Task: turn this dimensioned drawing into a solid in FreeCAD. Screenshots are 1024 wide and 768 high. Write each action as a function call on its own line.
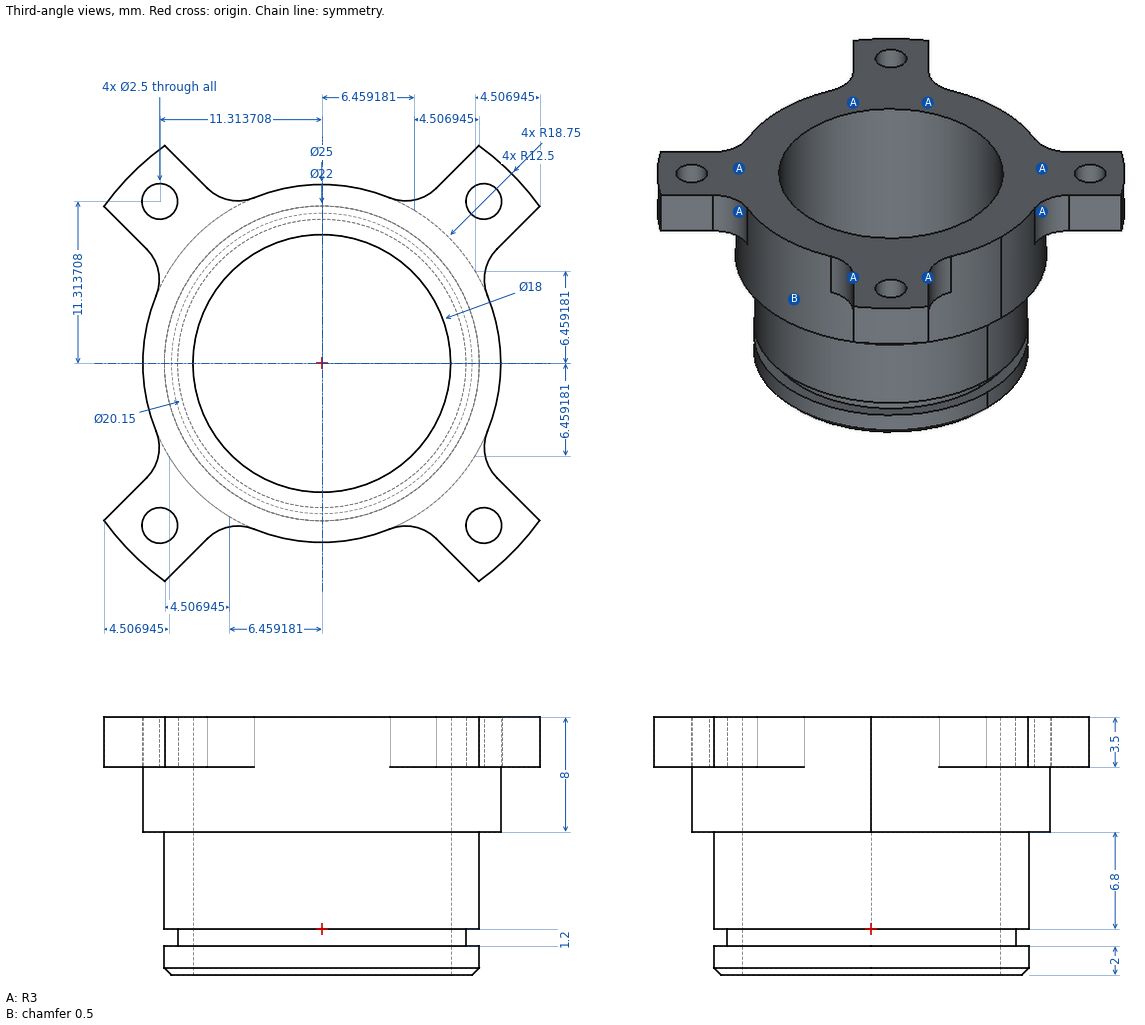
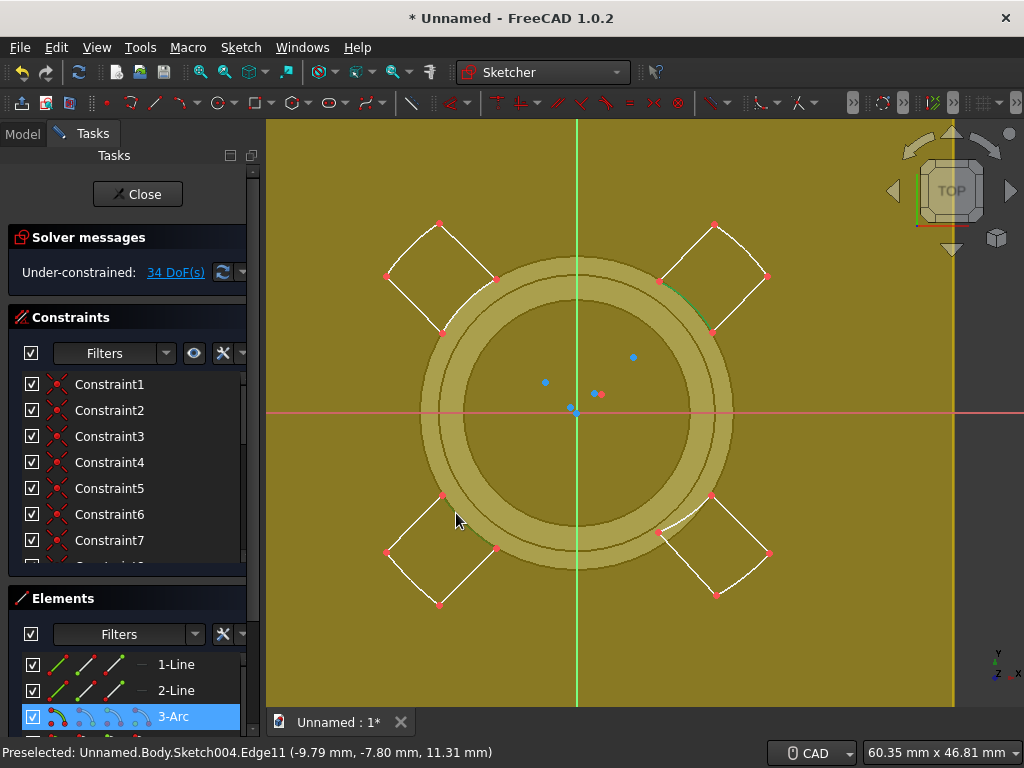
click(498, 104)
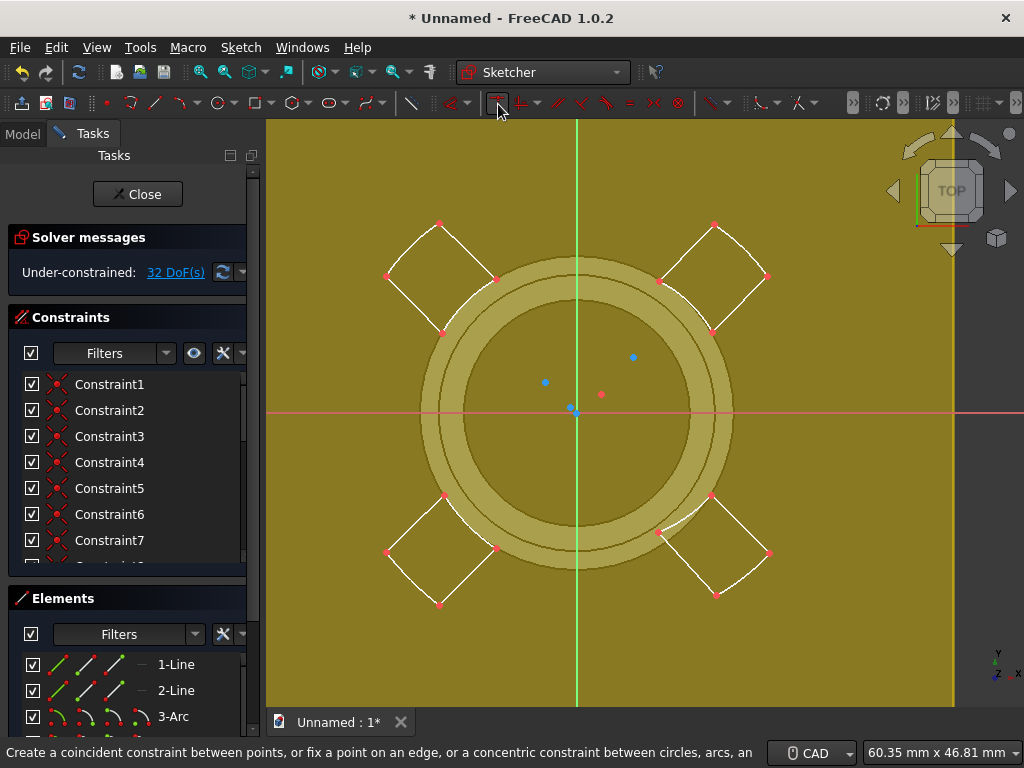
click(700, 314)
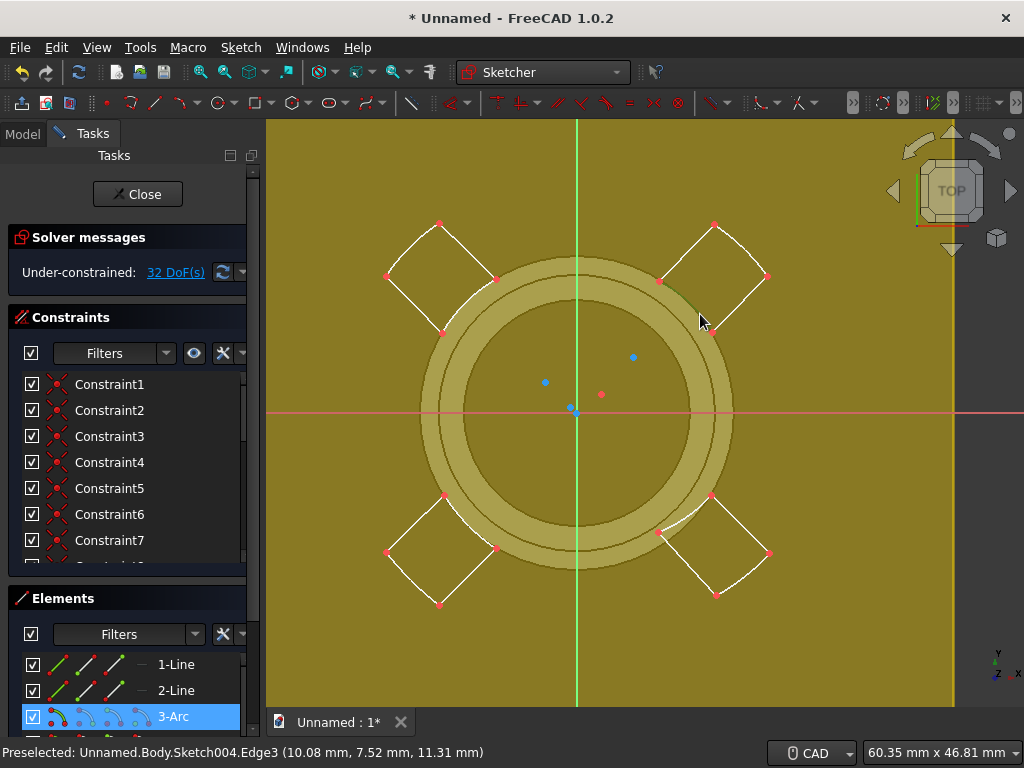
click(401, 569)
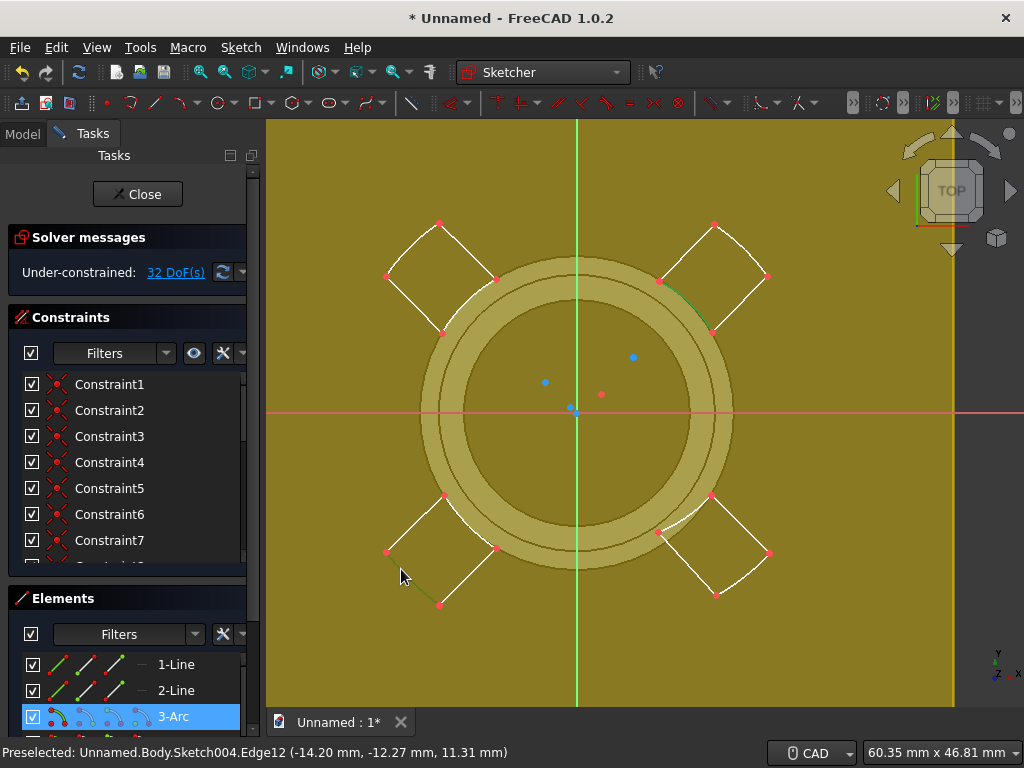
click(498, 104)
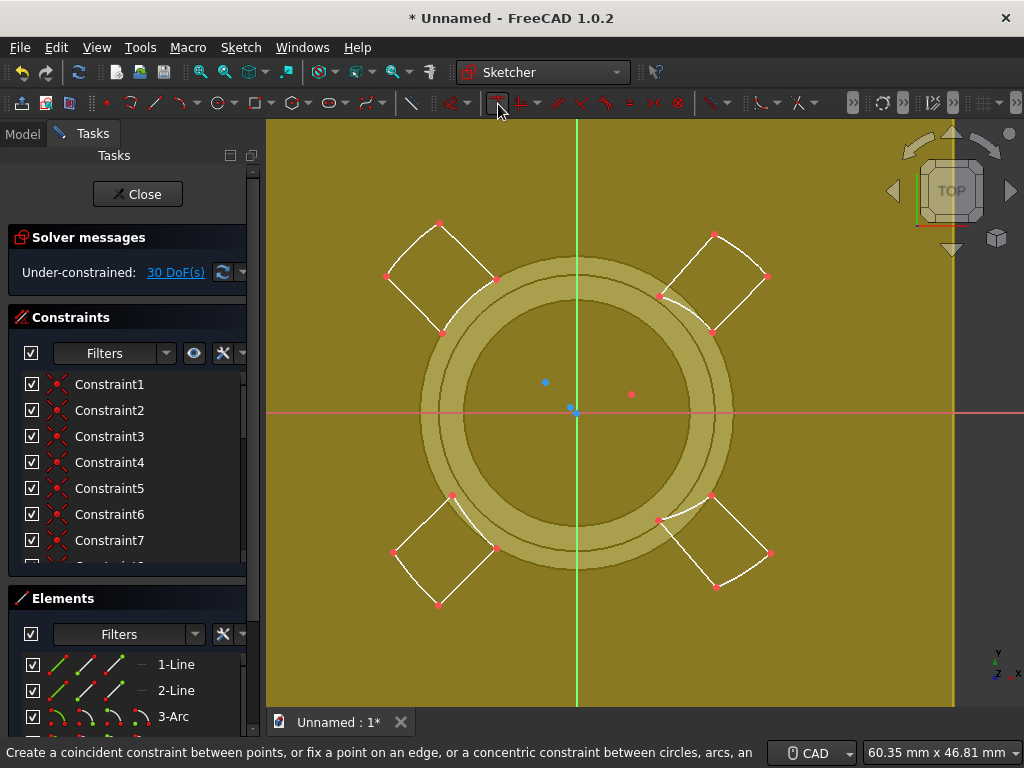
click(699, 318)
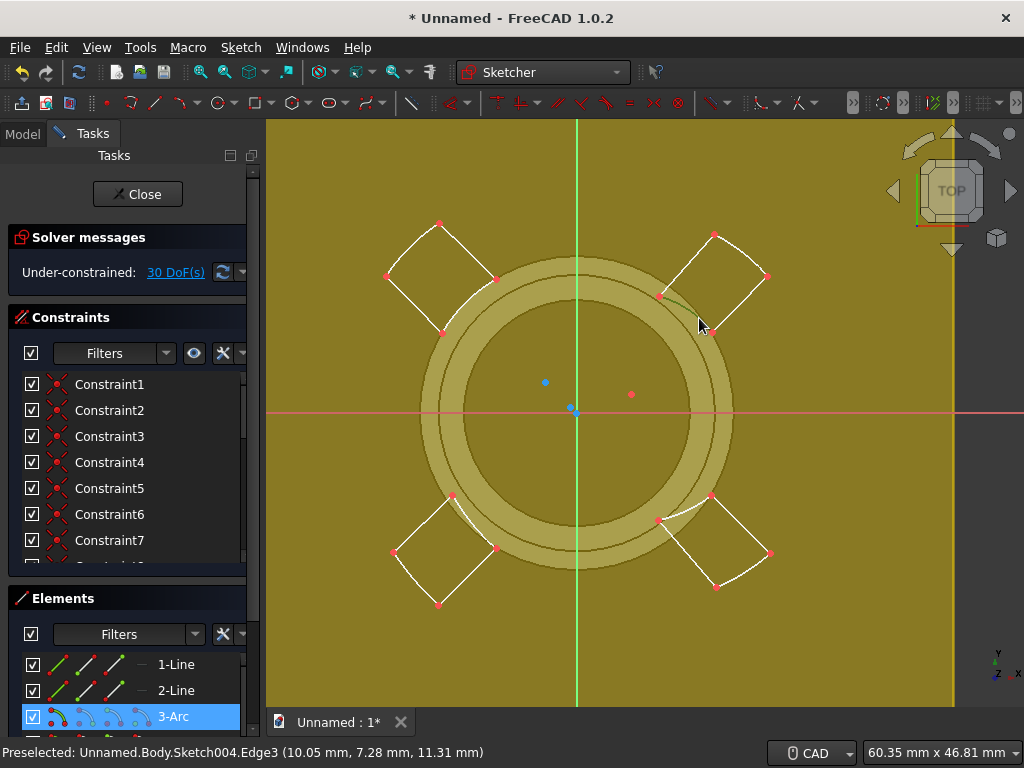
click(477, 292)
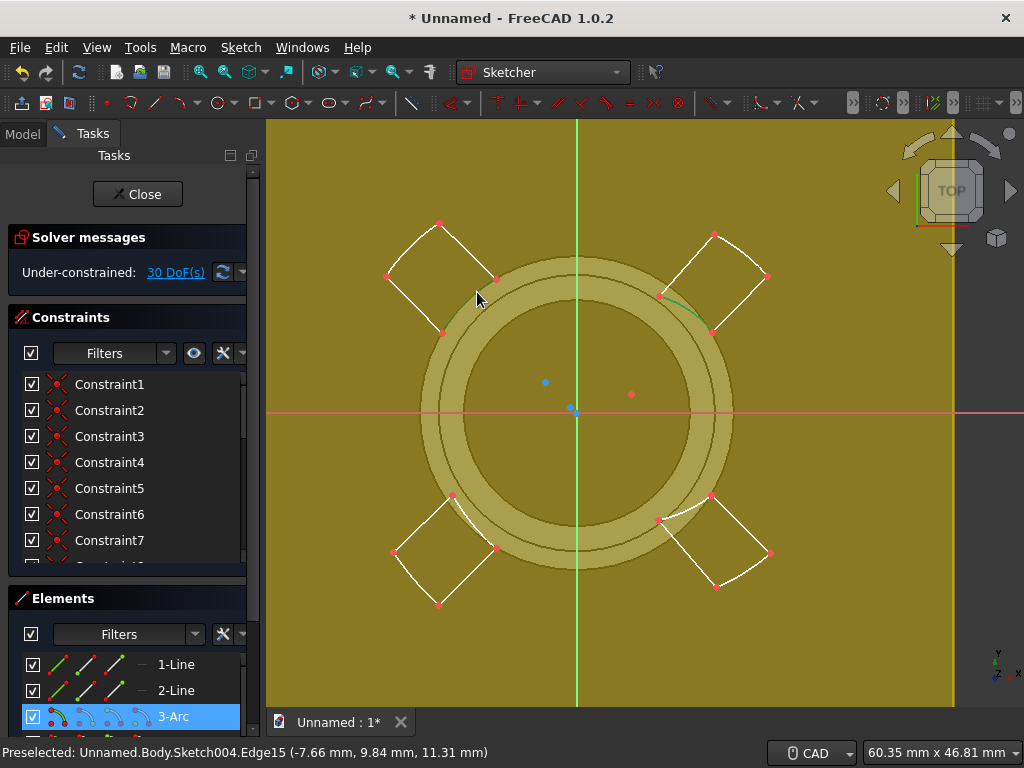
click(498, 104)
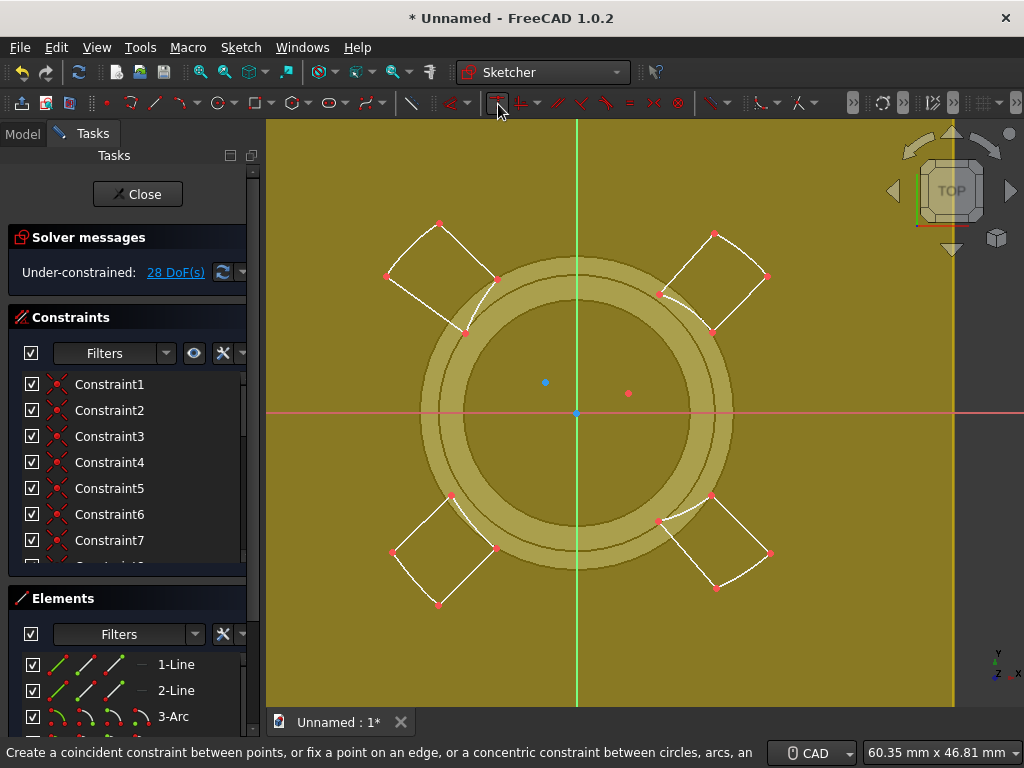
click(699, 317)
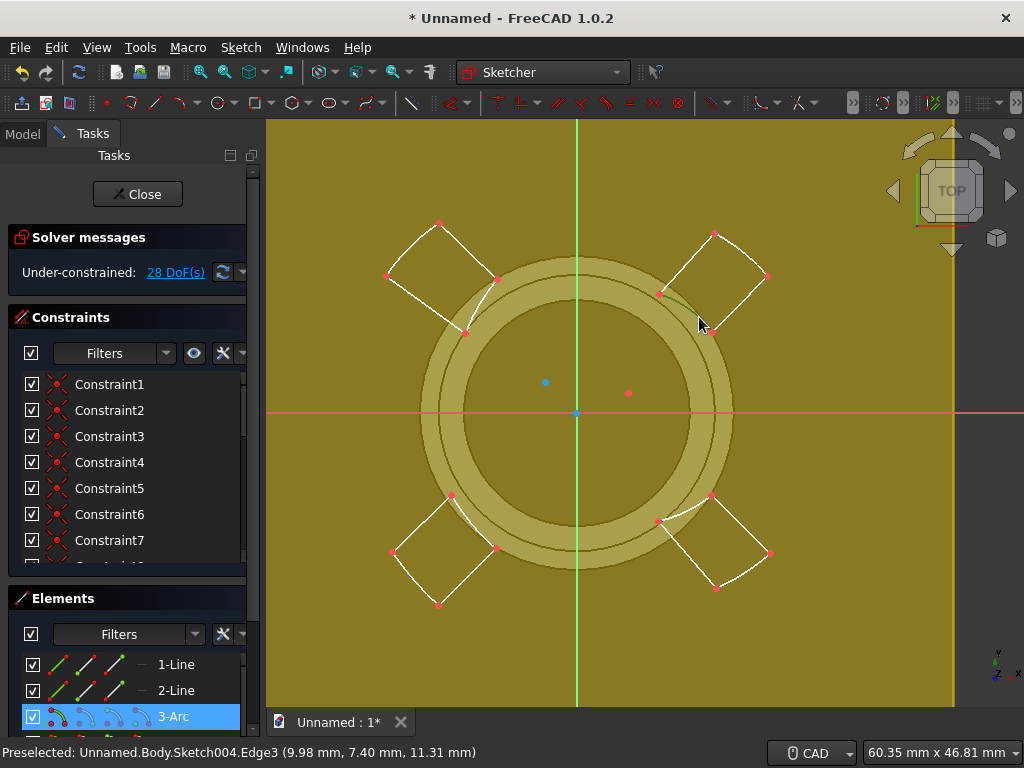
click(421, 237)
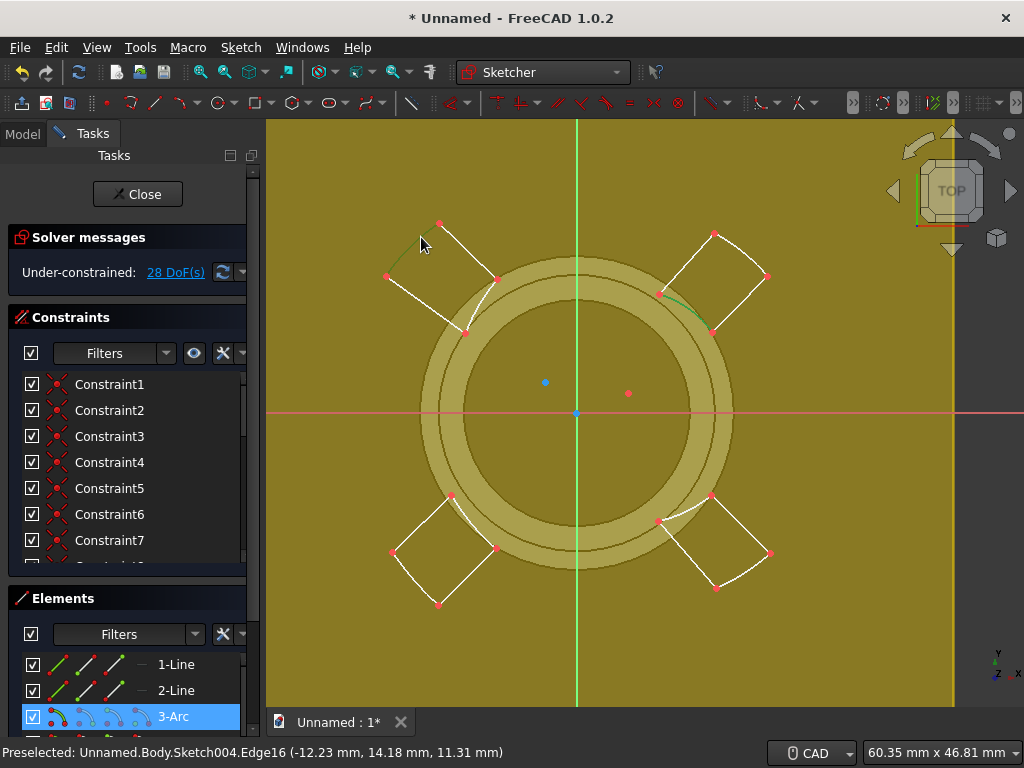
click(498, 104)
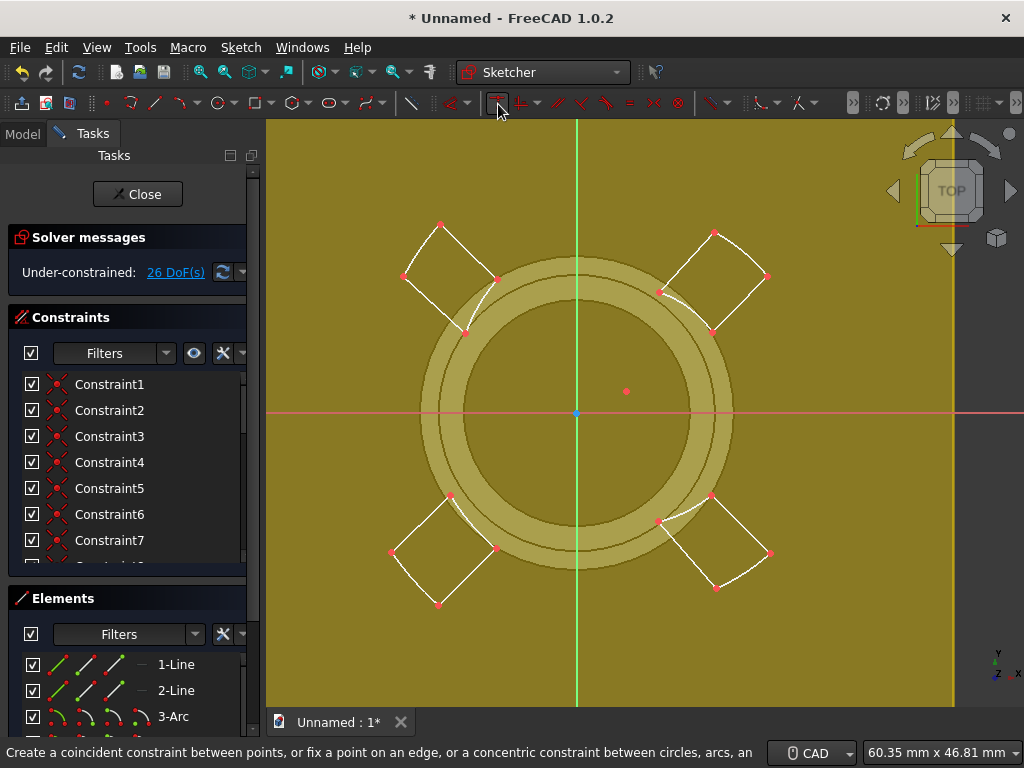
drag(567, 382, 636, 423)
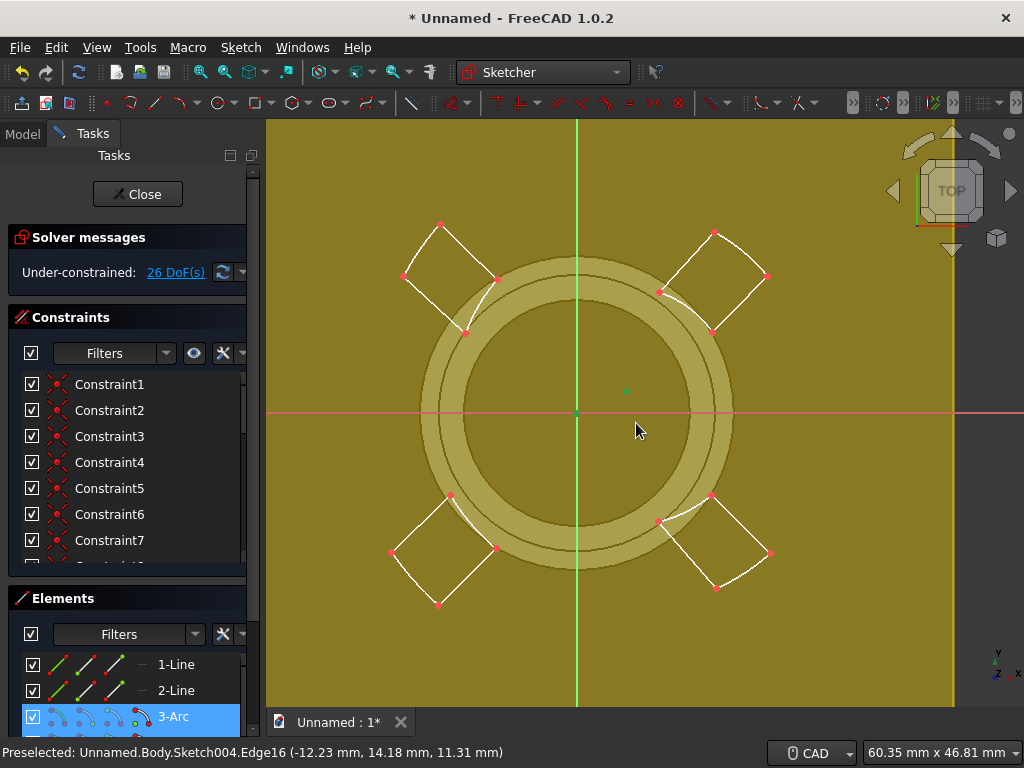
click(498, 104)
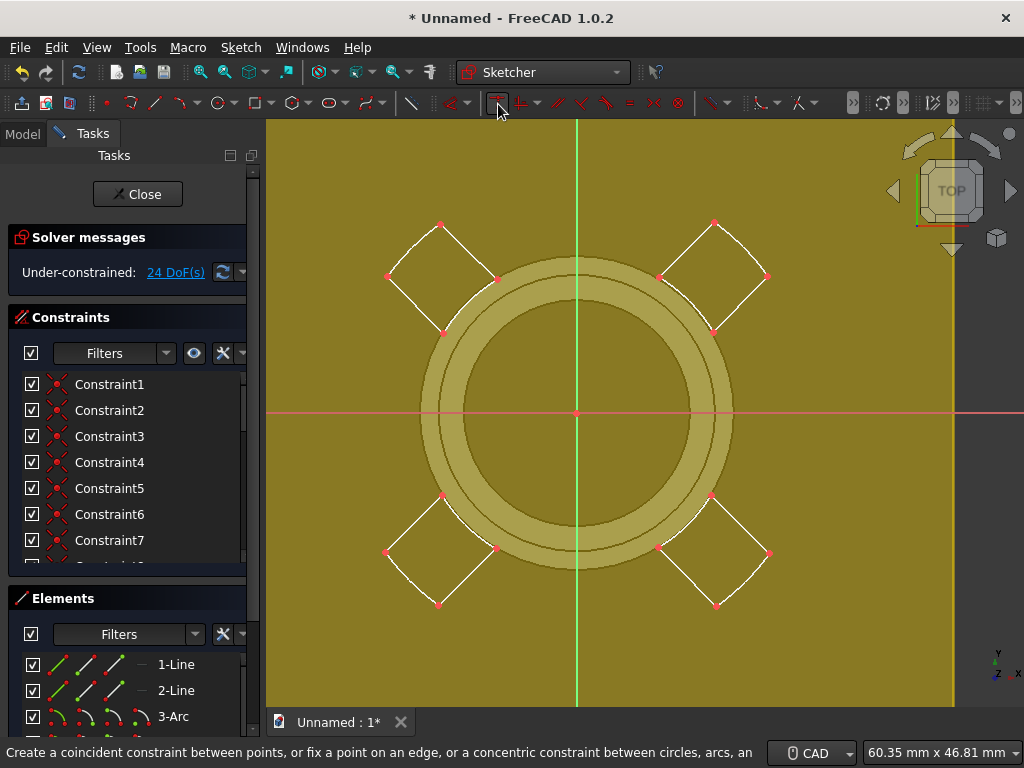
click(700, 313)